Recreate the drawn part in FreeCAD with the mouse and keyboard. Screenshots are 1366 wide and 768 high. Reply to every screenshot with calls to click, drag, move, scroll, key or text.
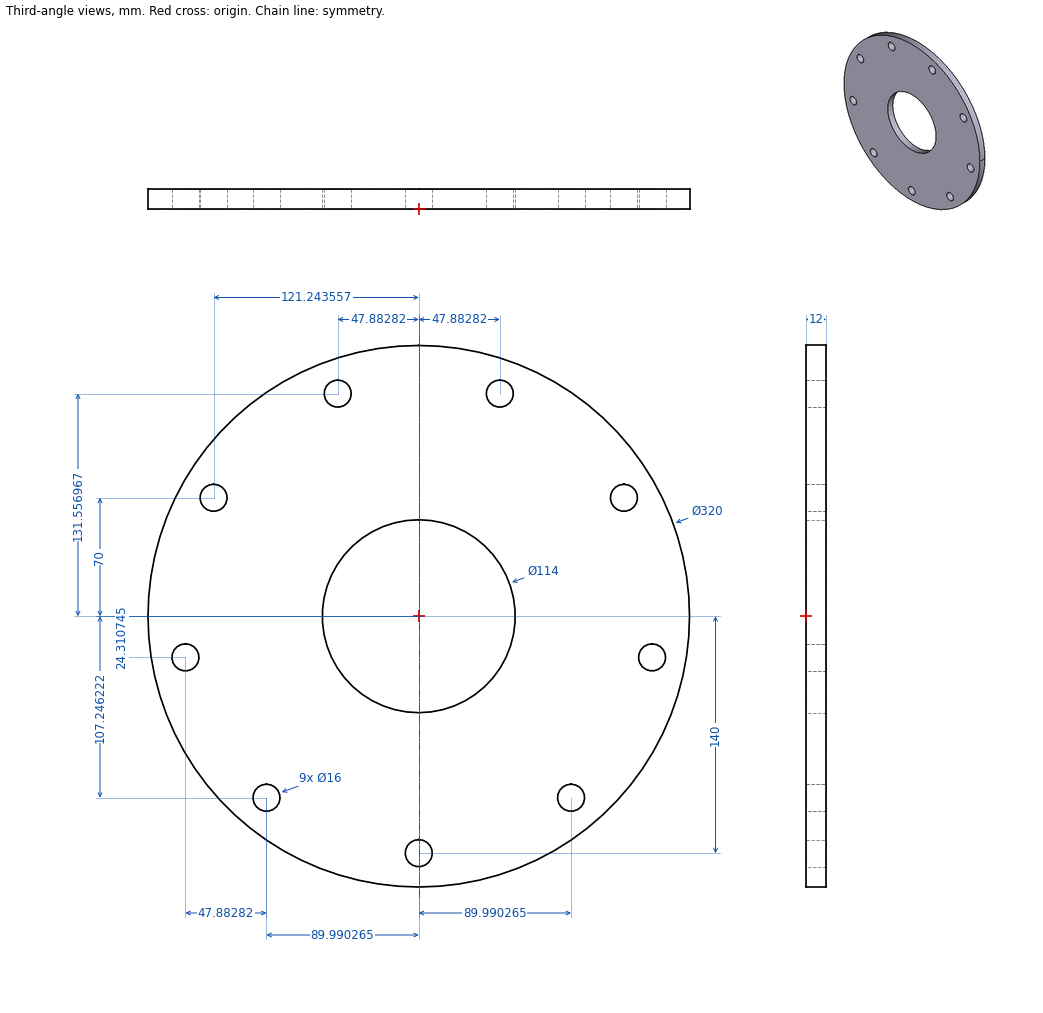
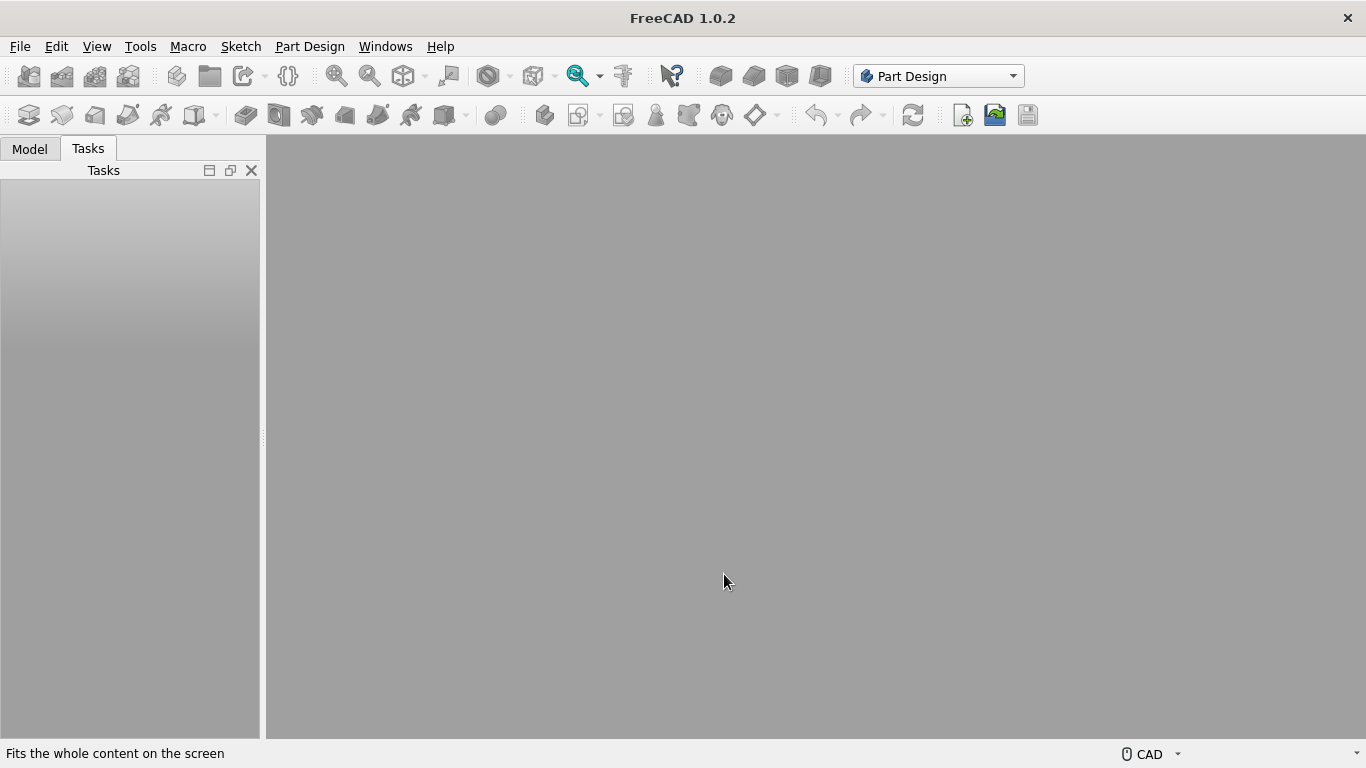
click(962, 116)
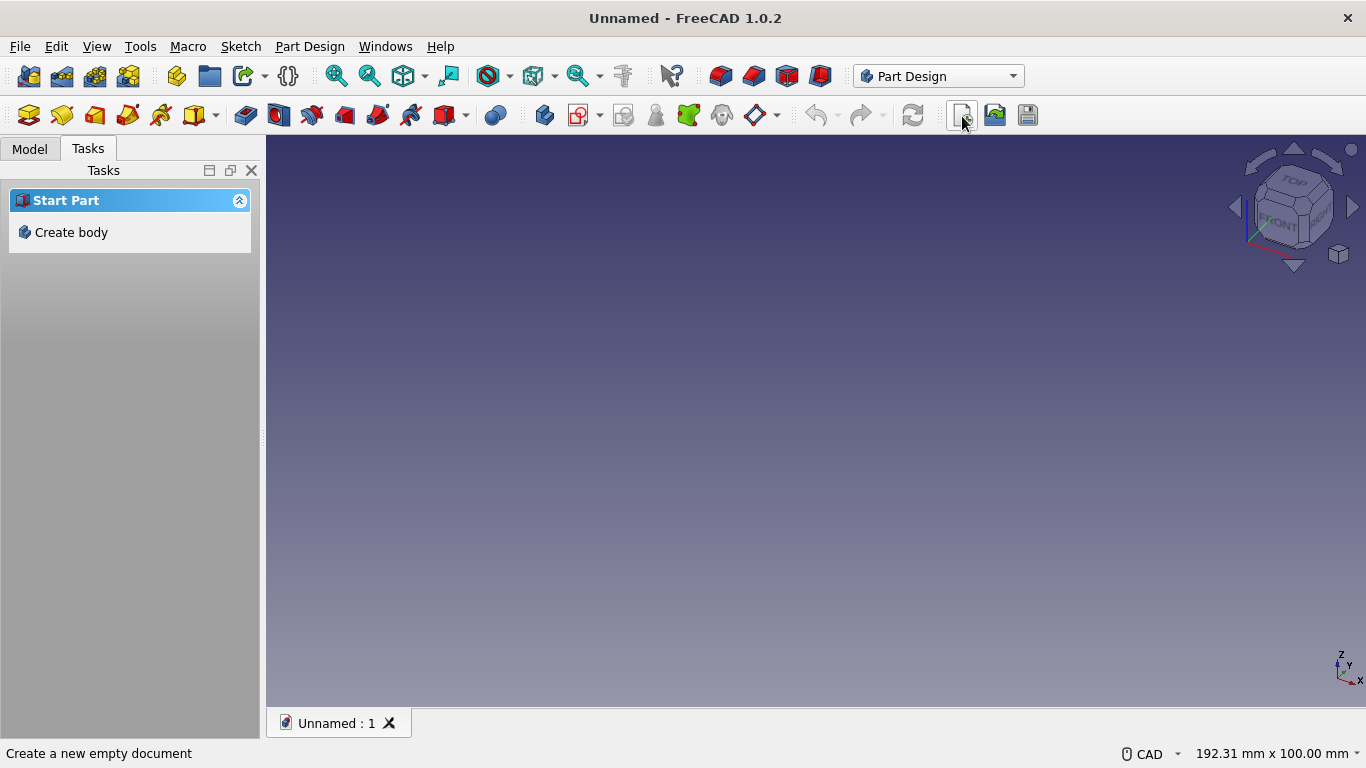
click(578, 116)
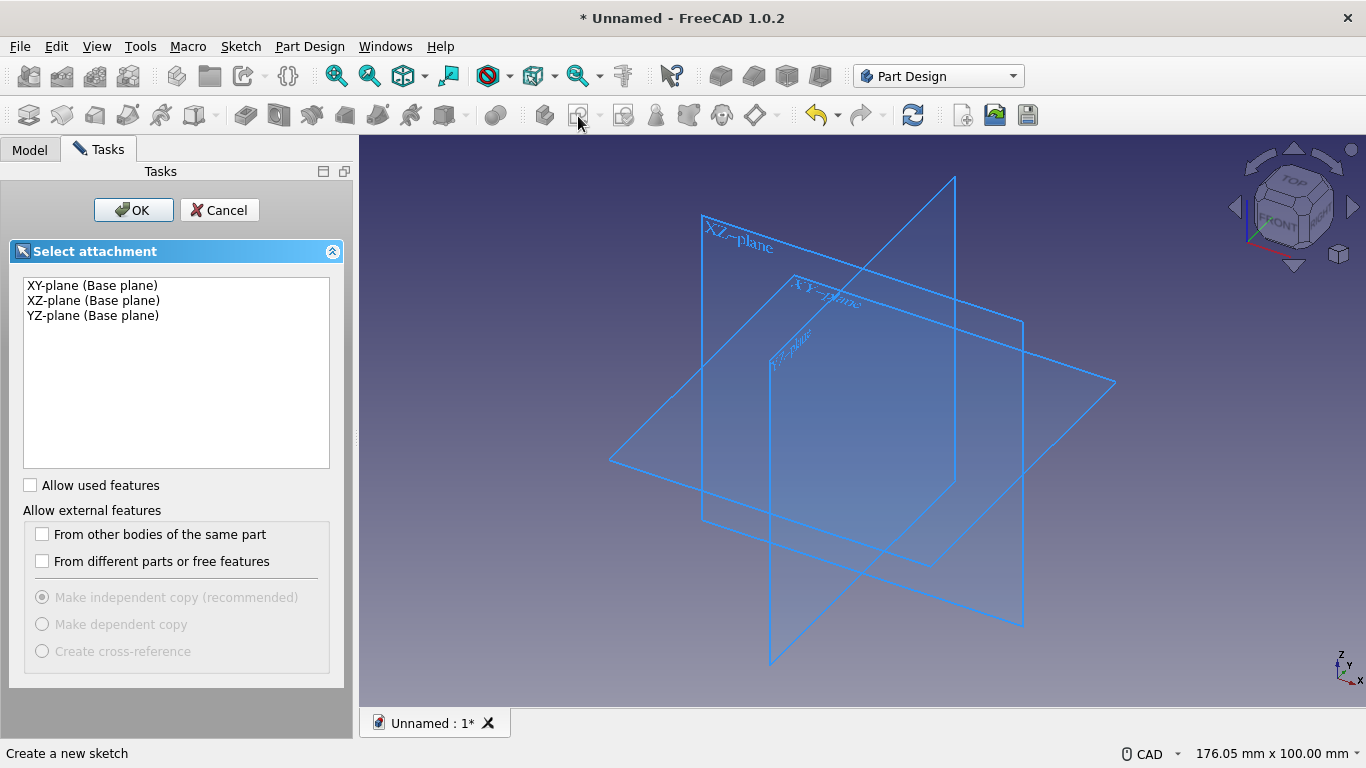
click(84, 300)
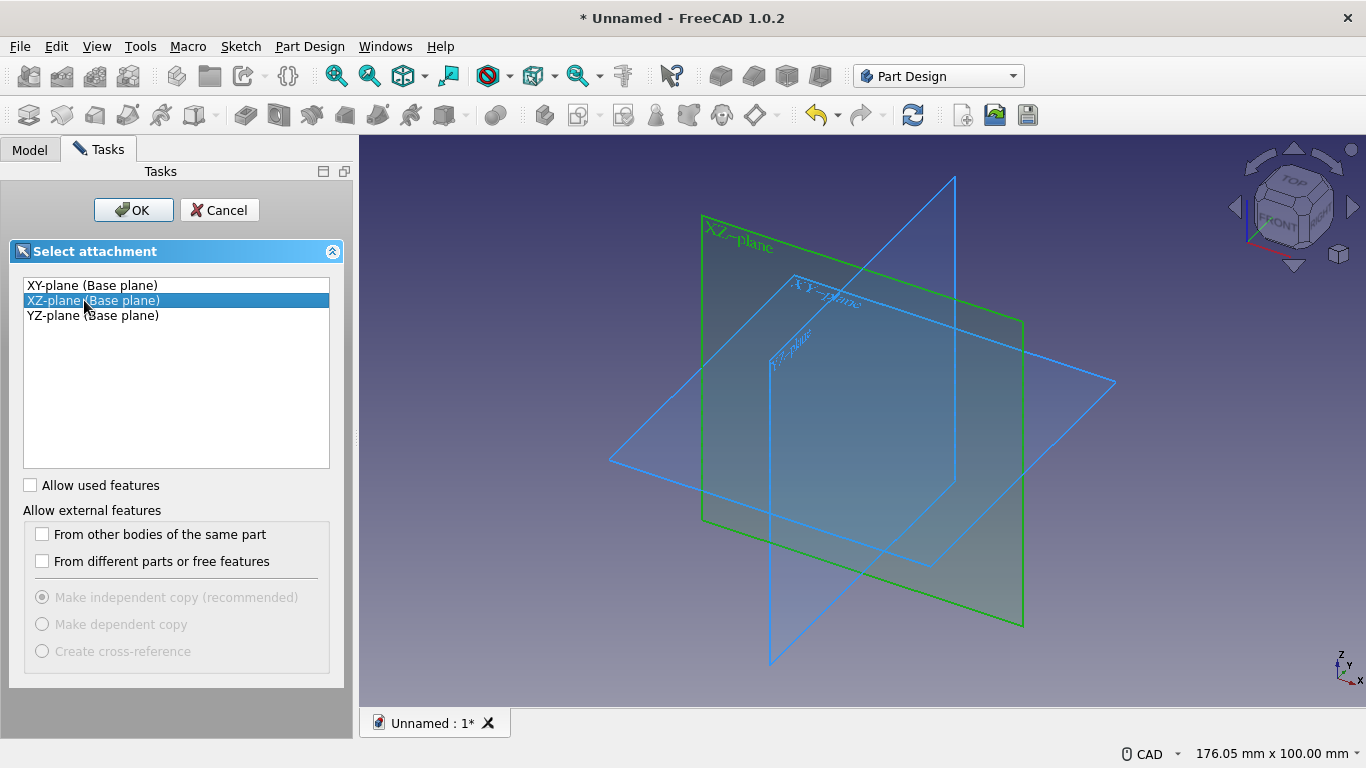
click(134, 210)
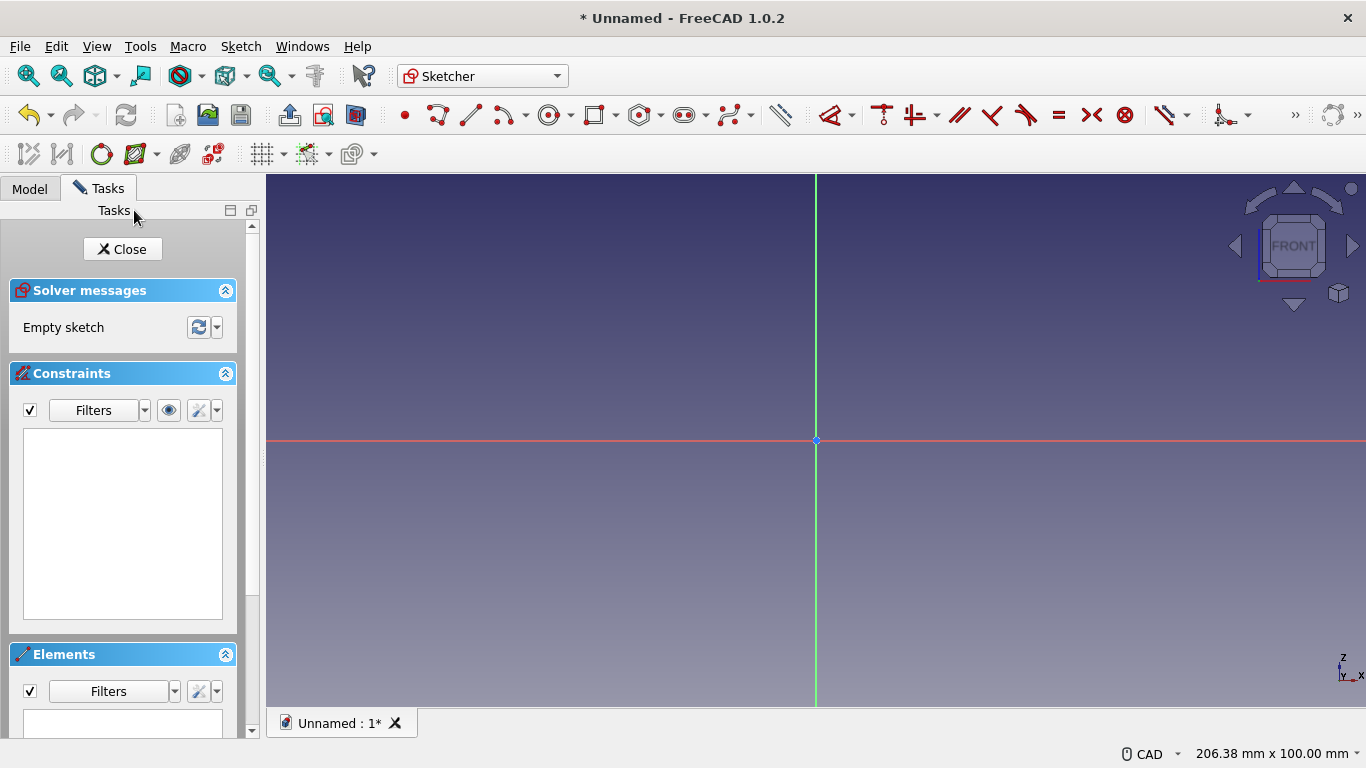
scroll(730, 440, down, 8)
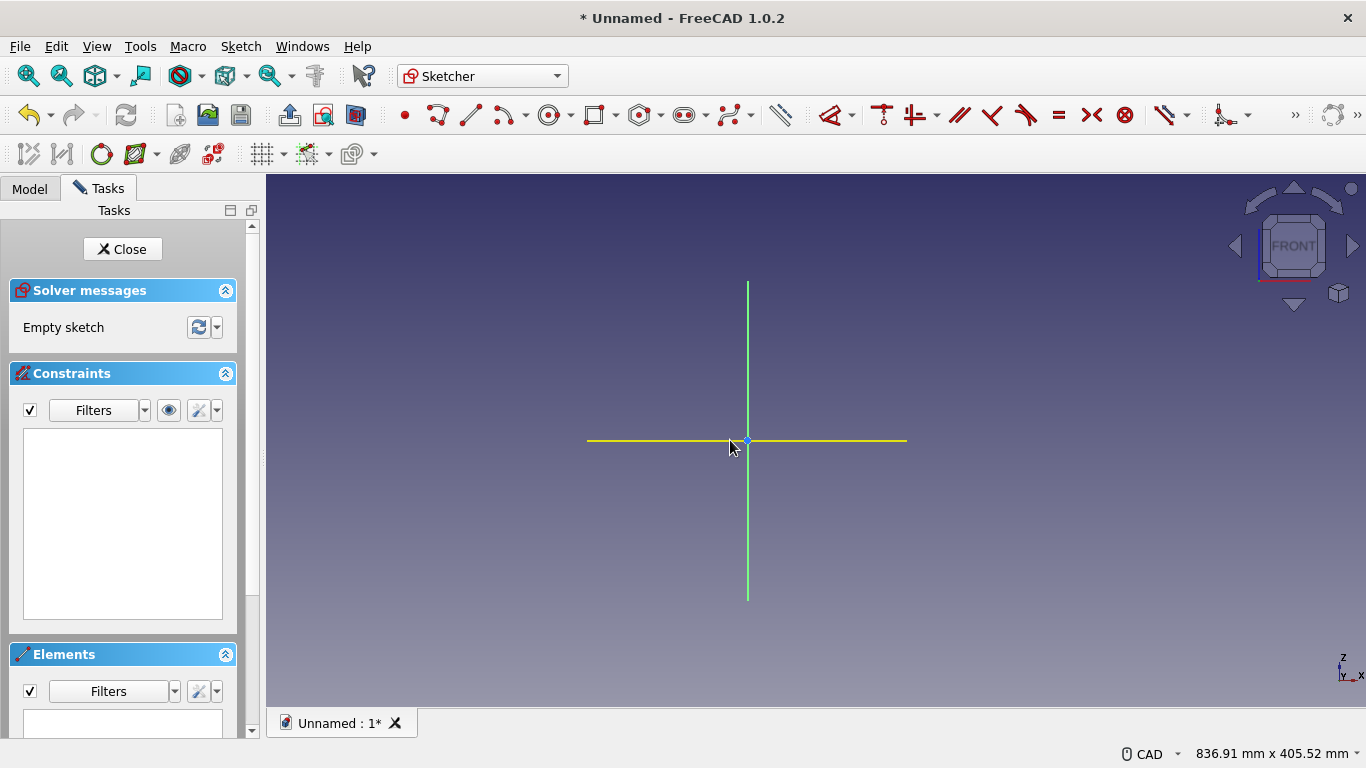
click(548, 116)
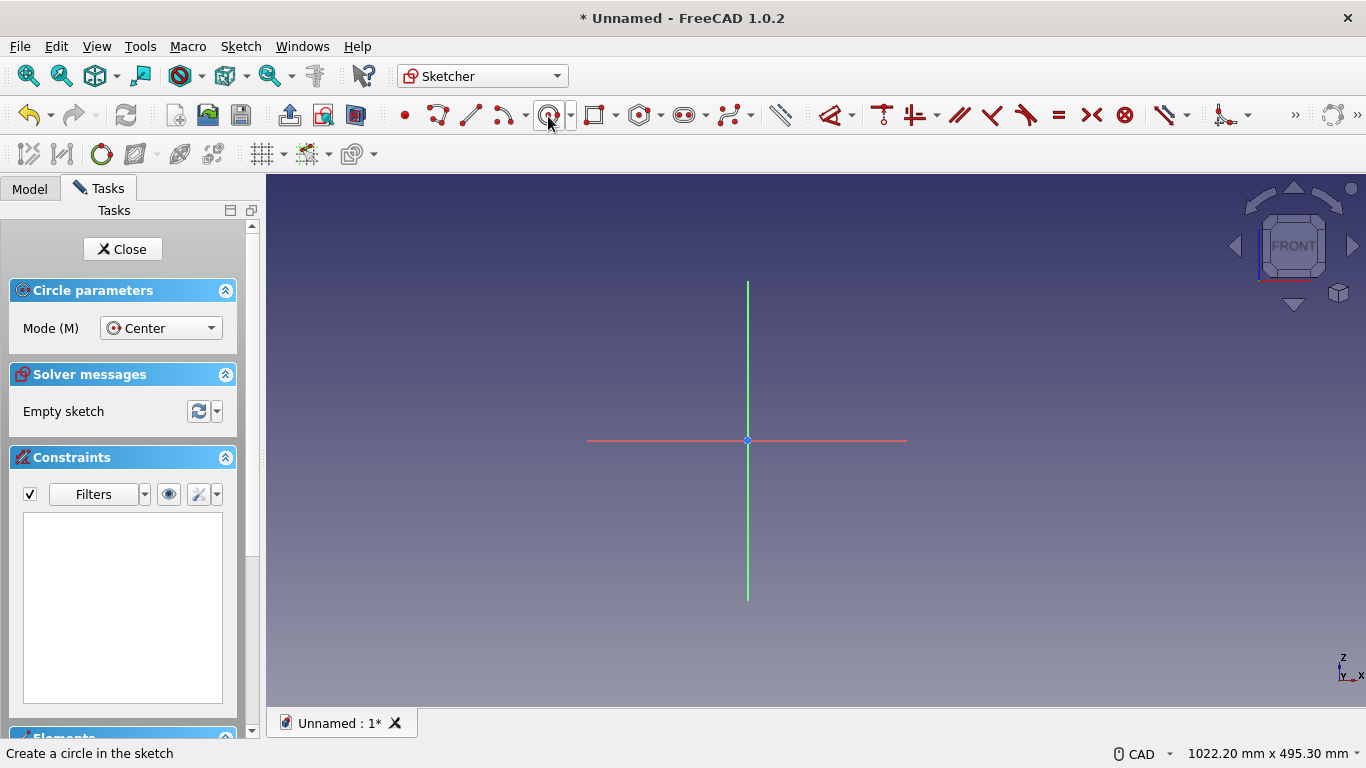
click(748, 440)
move(869, 319)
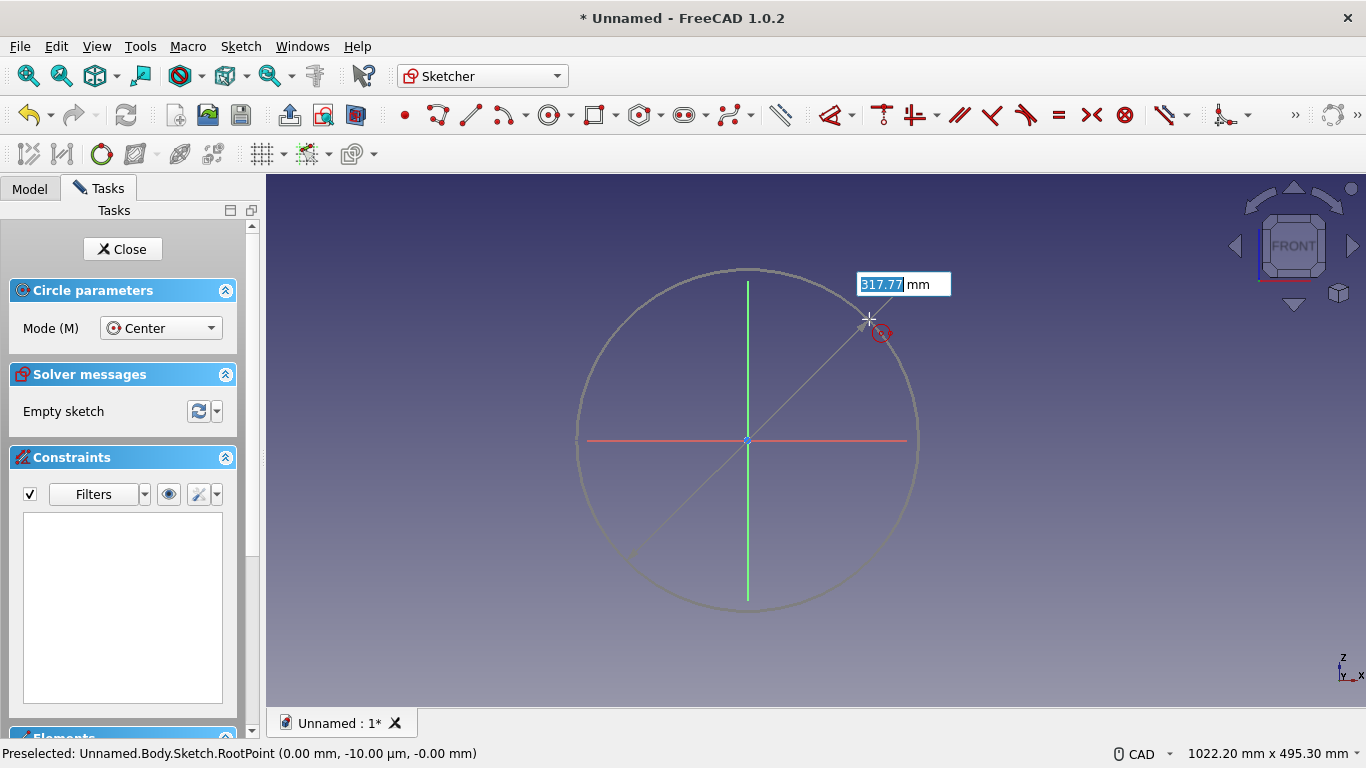
text(320)
key(Return)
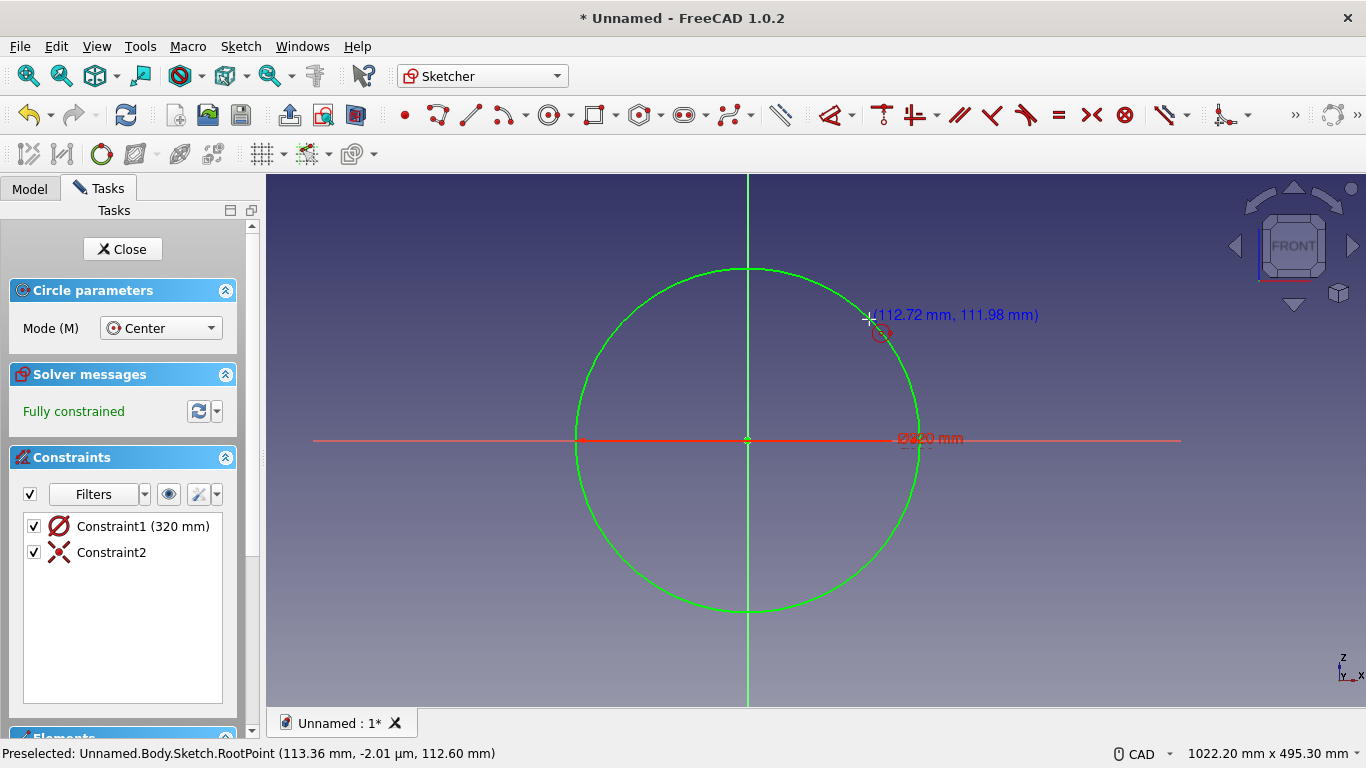
scroll(651, 556, up, 5)